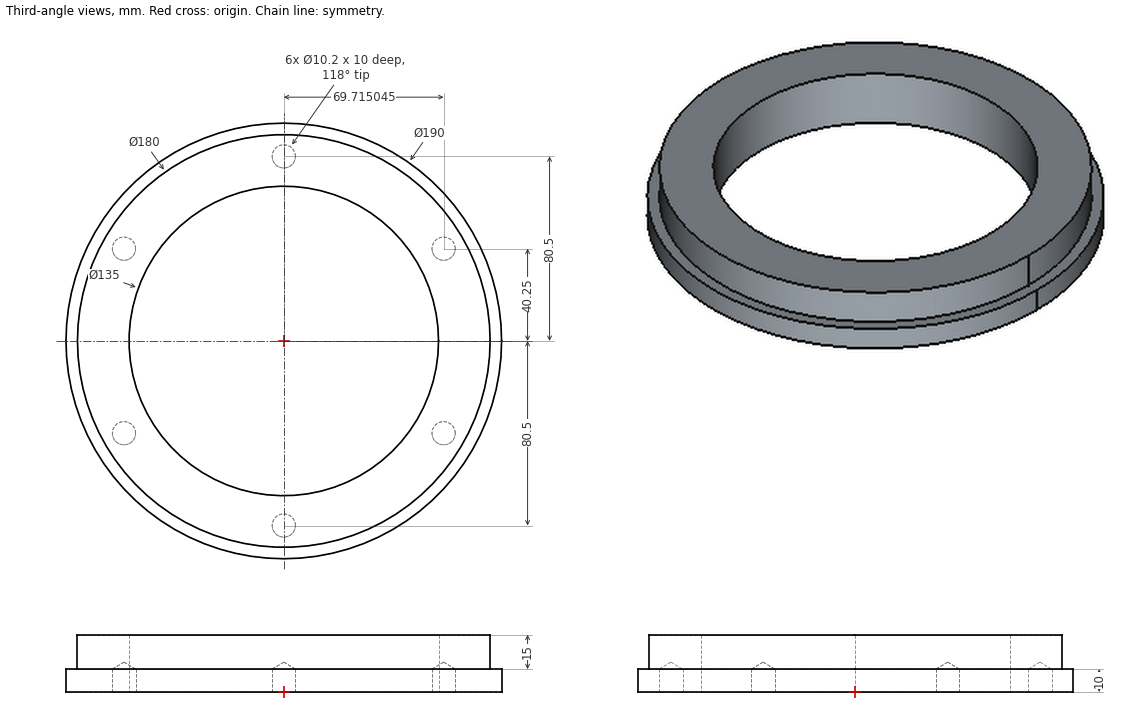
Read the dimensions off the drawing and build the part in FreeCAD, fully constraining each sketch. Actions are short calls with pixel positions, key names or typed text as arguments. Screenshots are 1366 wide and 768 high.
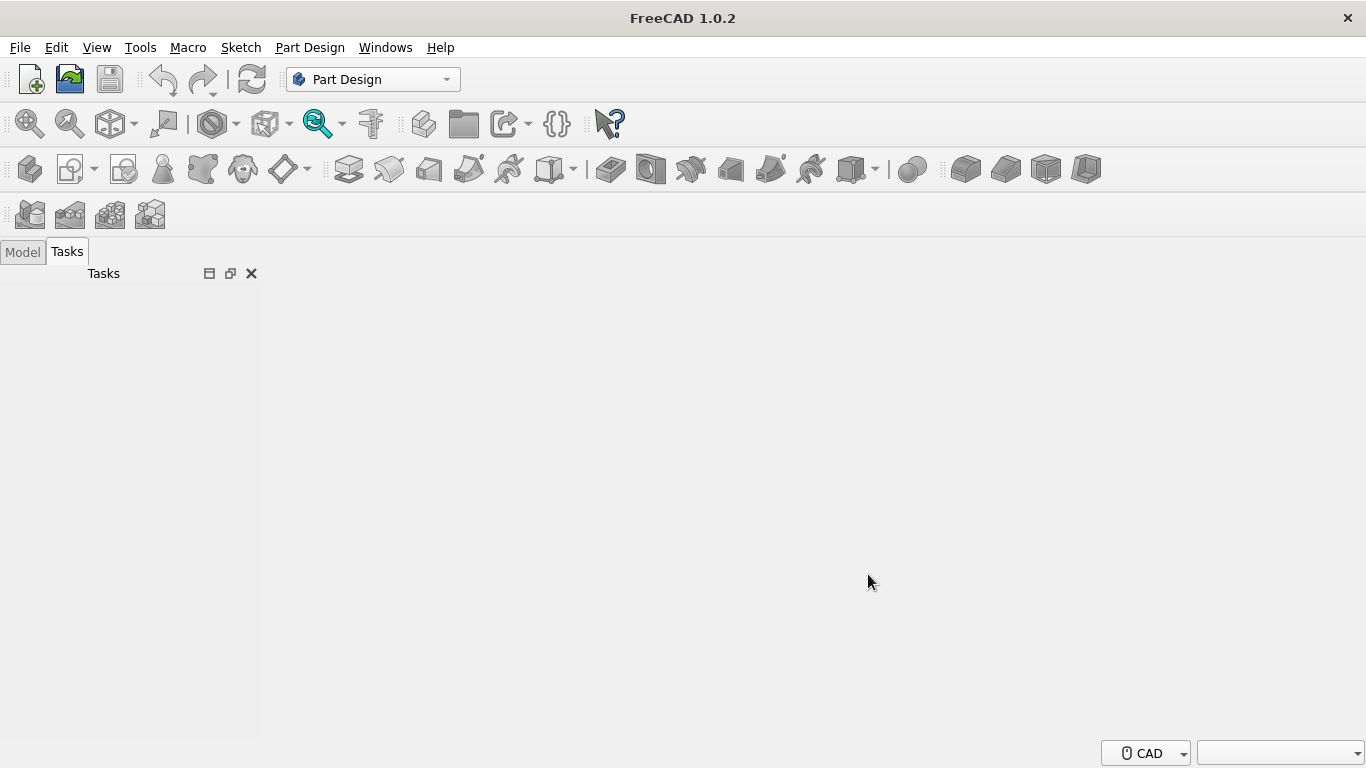
key(ctrl+n)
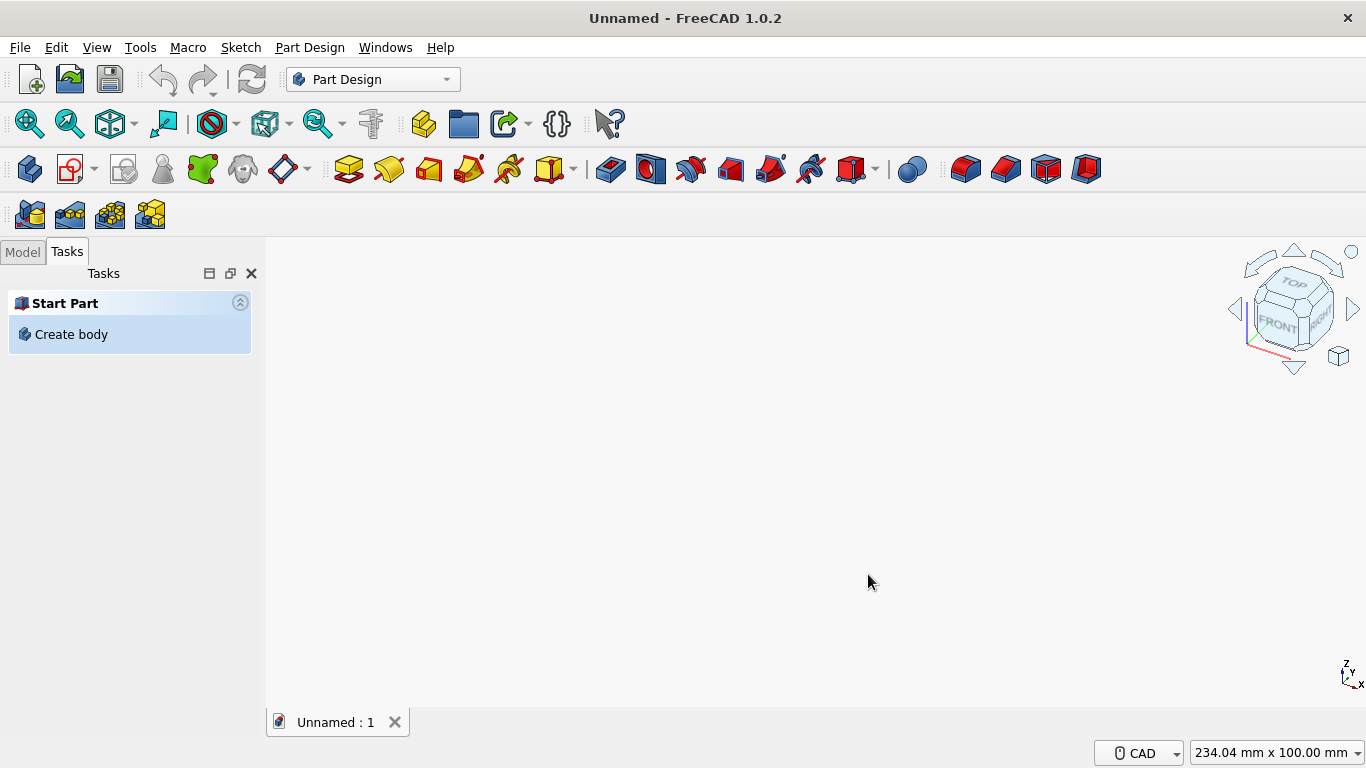
click(70, 170)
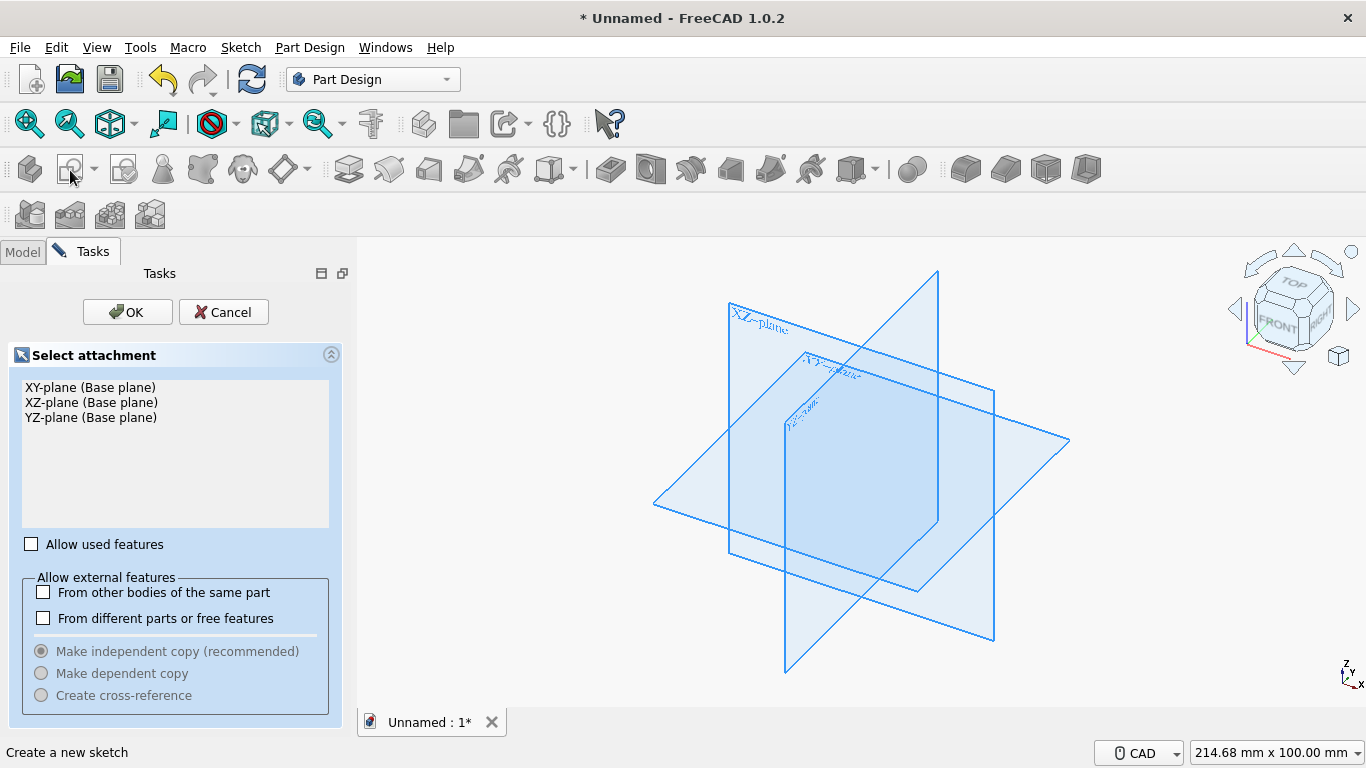
click(82, 388)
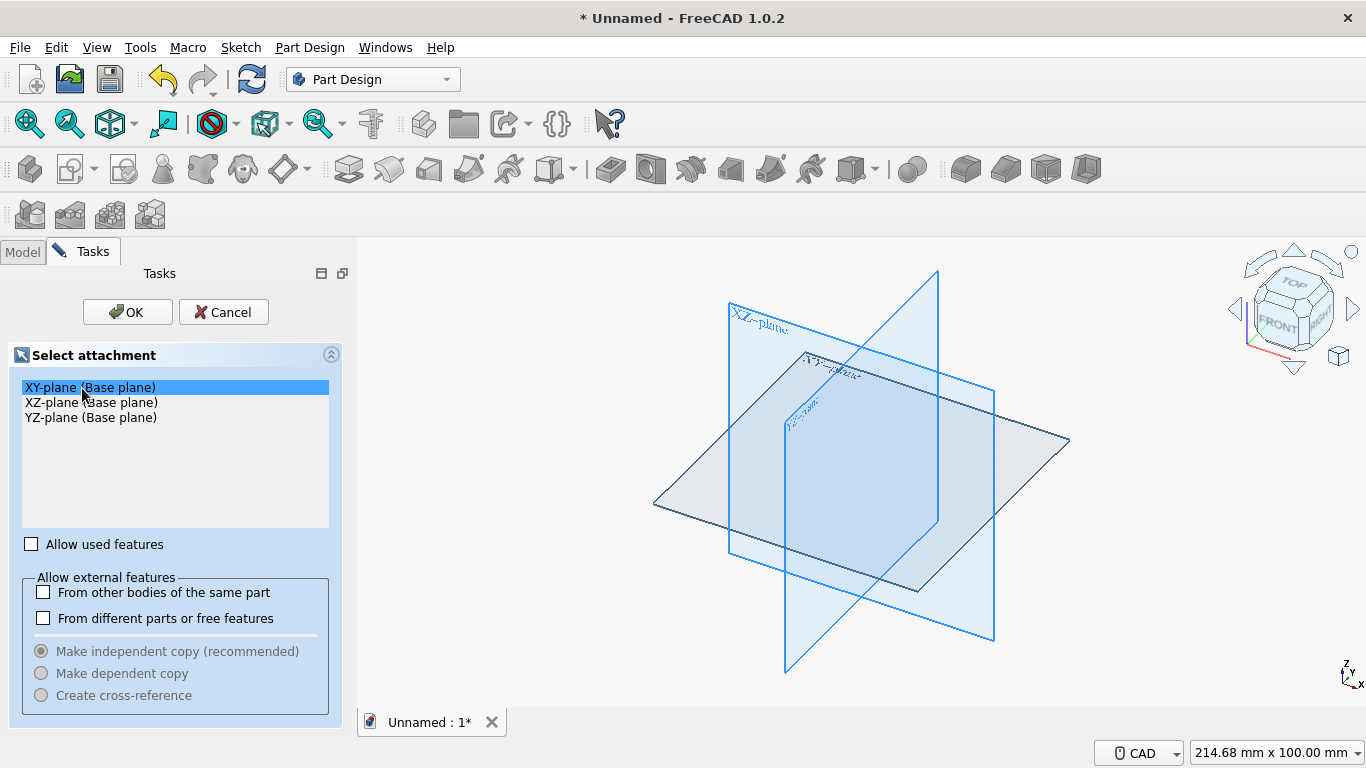
click(128, 312)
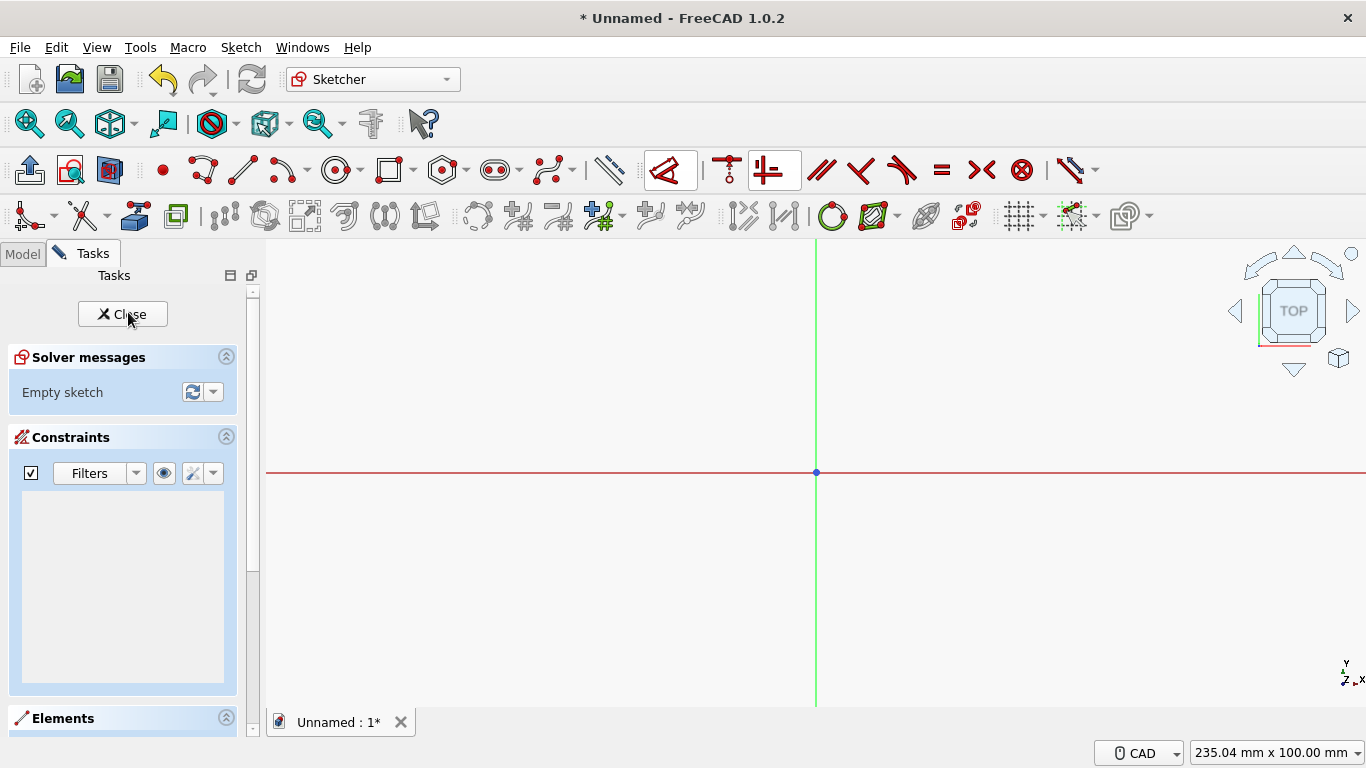
scroll(718, 473, down, 6)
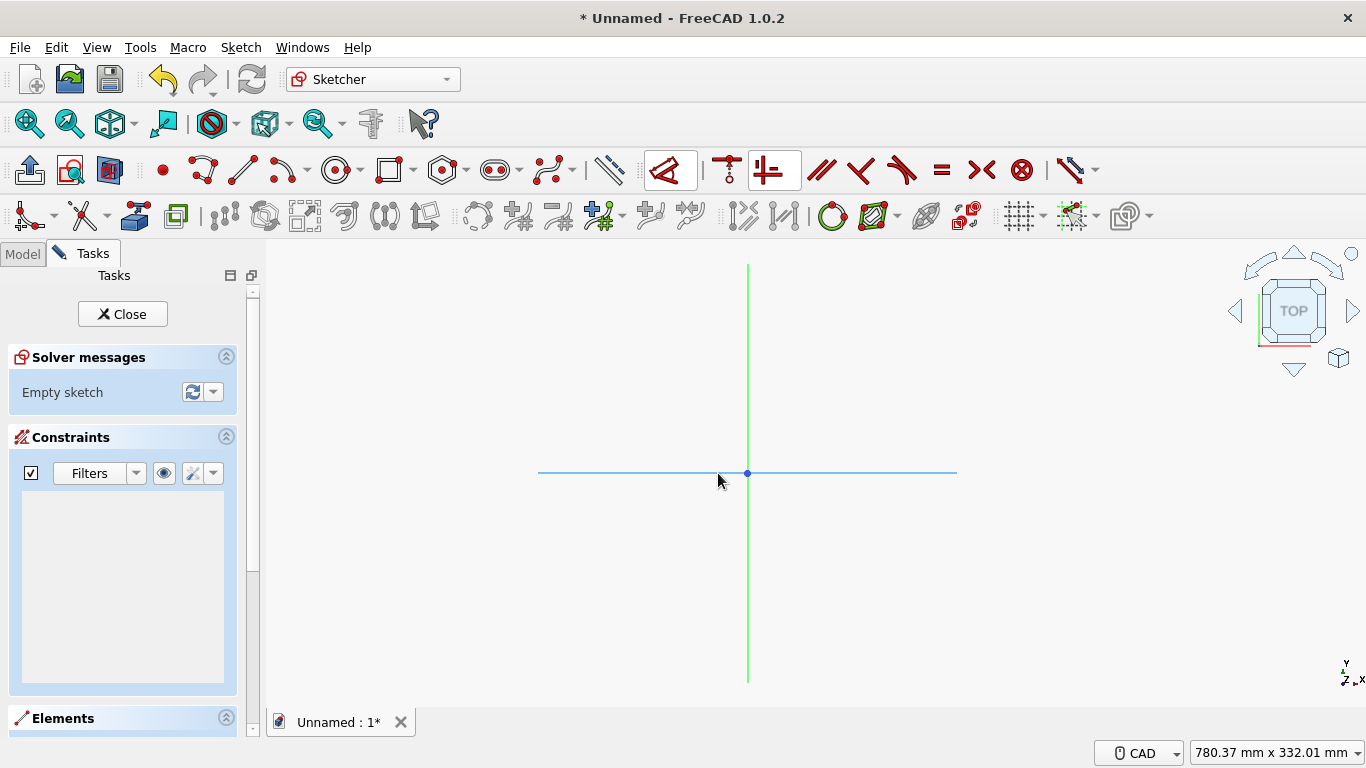
key(g)
key(c)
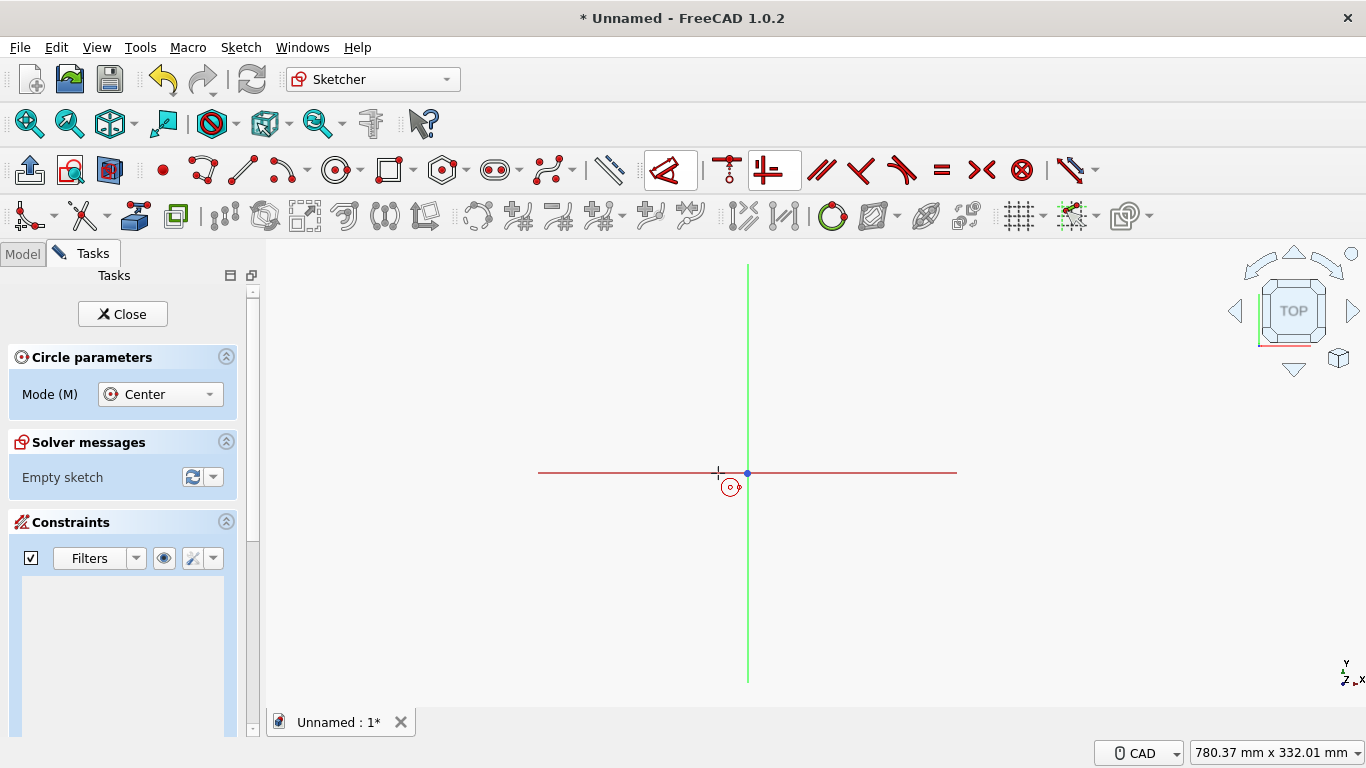
click(748, 473)
move(842, 379)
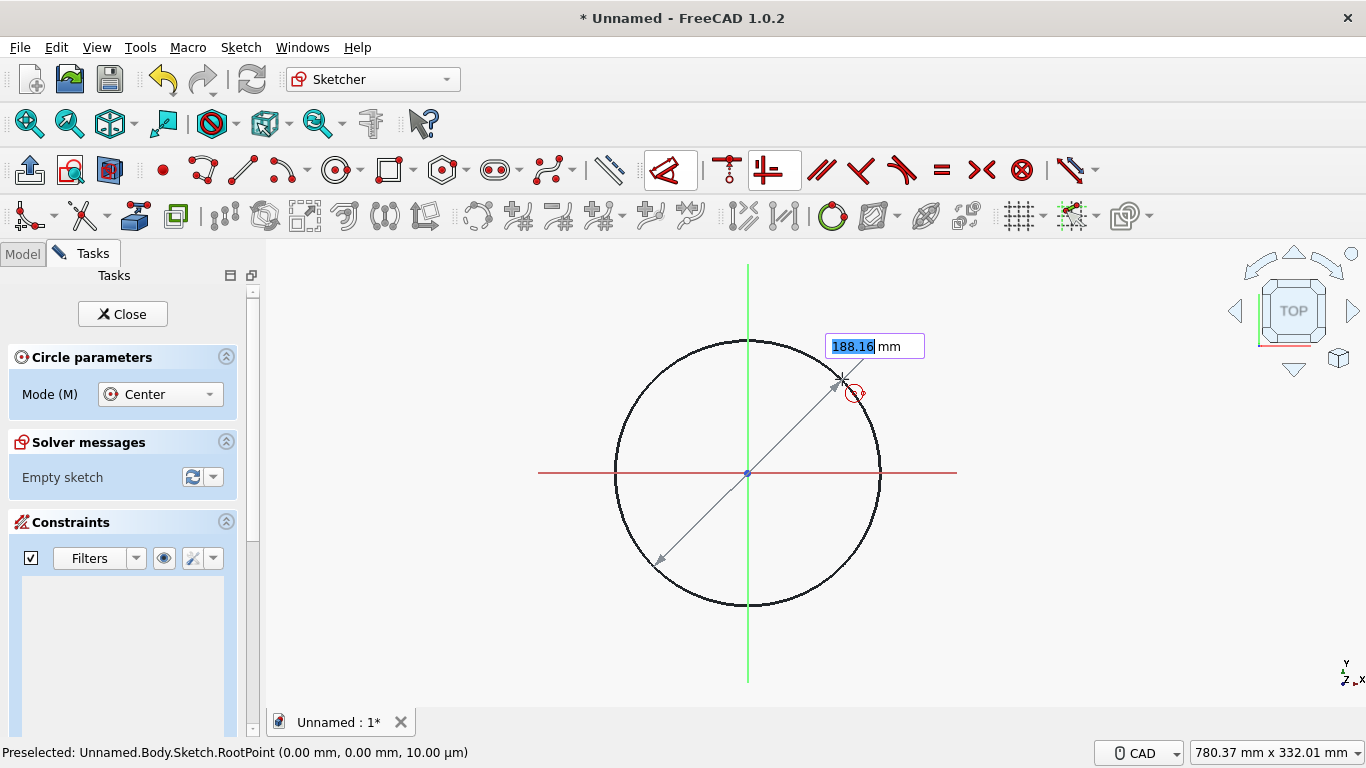
text(190)
key(Return)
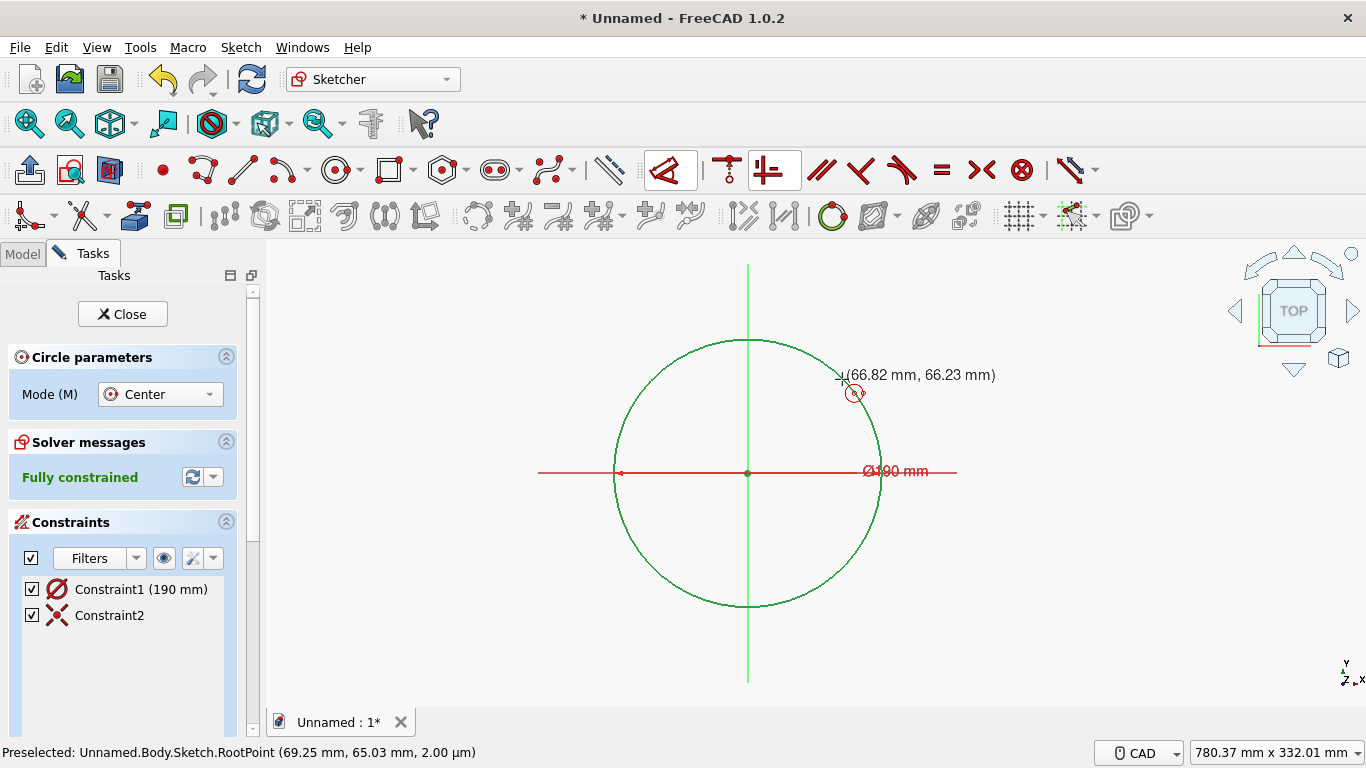
click(748, 473)
move(815, 406)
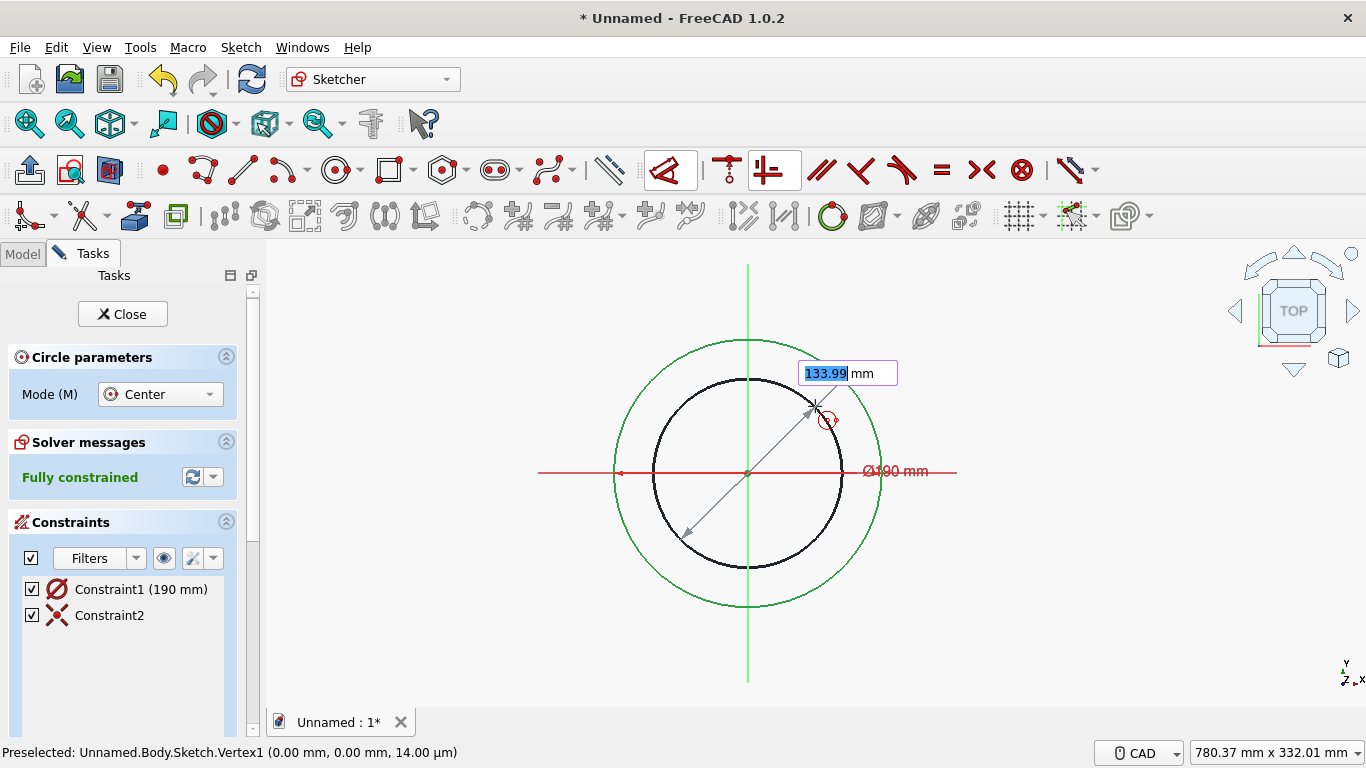
text(135)
key(Return)
key(Escape)